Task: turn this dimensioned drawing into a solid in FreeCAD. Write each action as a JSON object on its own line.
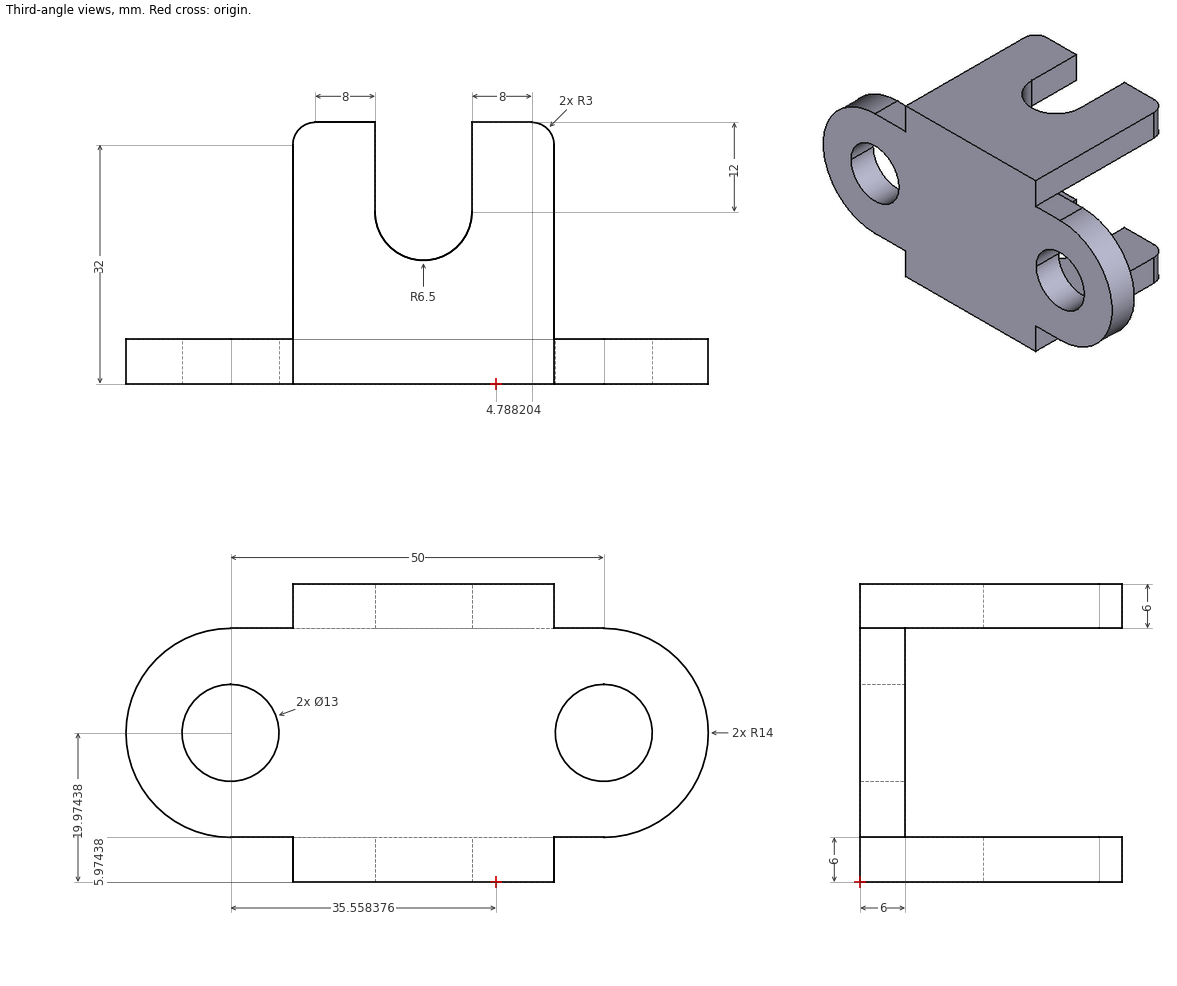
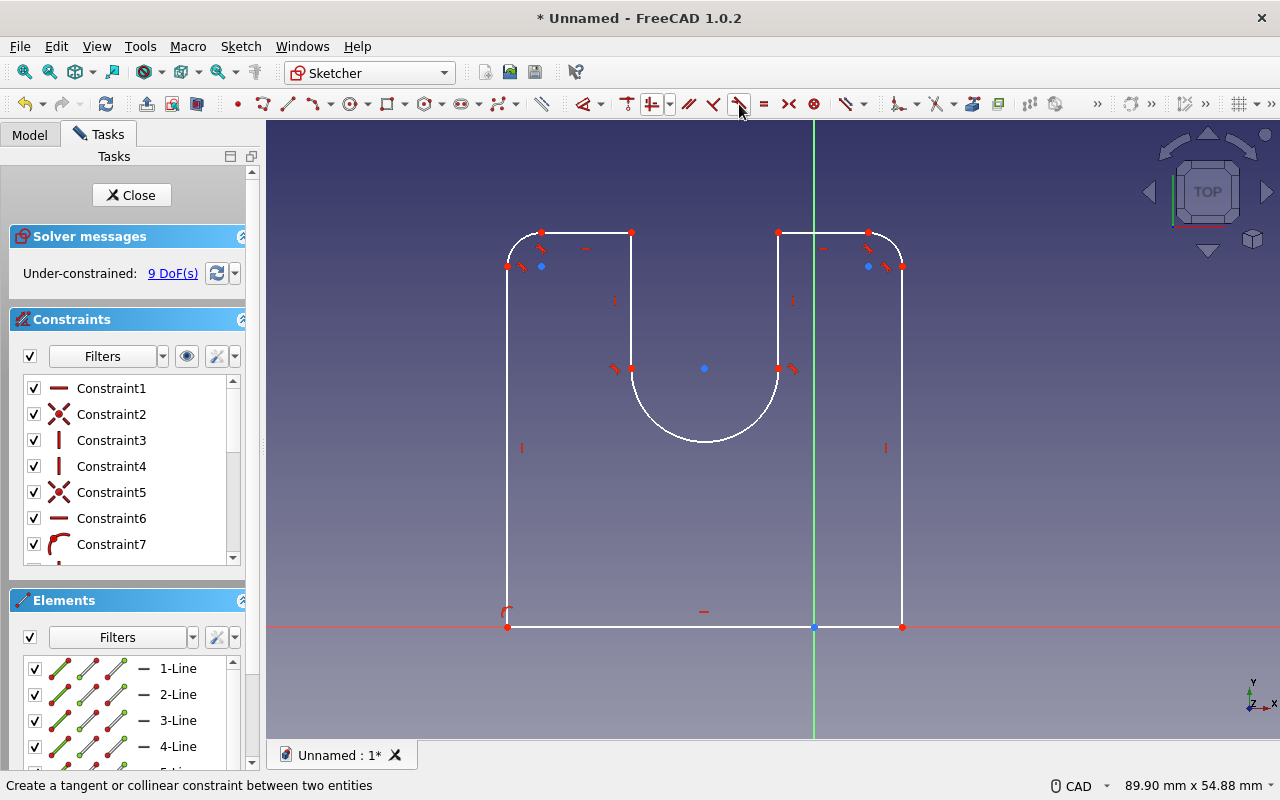
{"action": "left_click", "coordinate": [526, 237]}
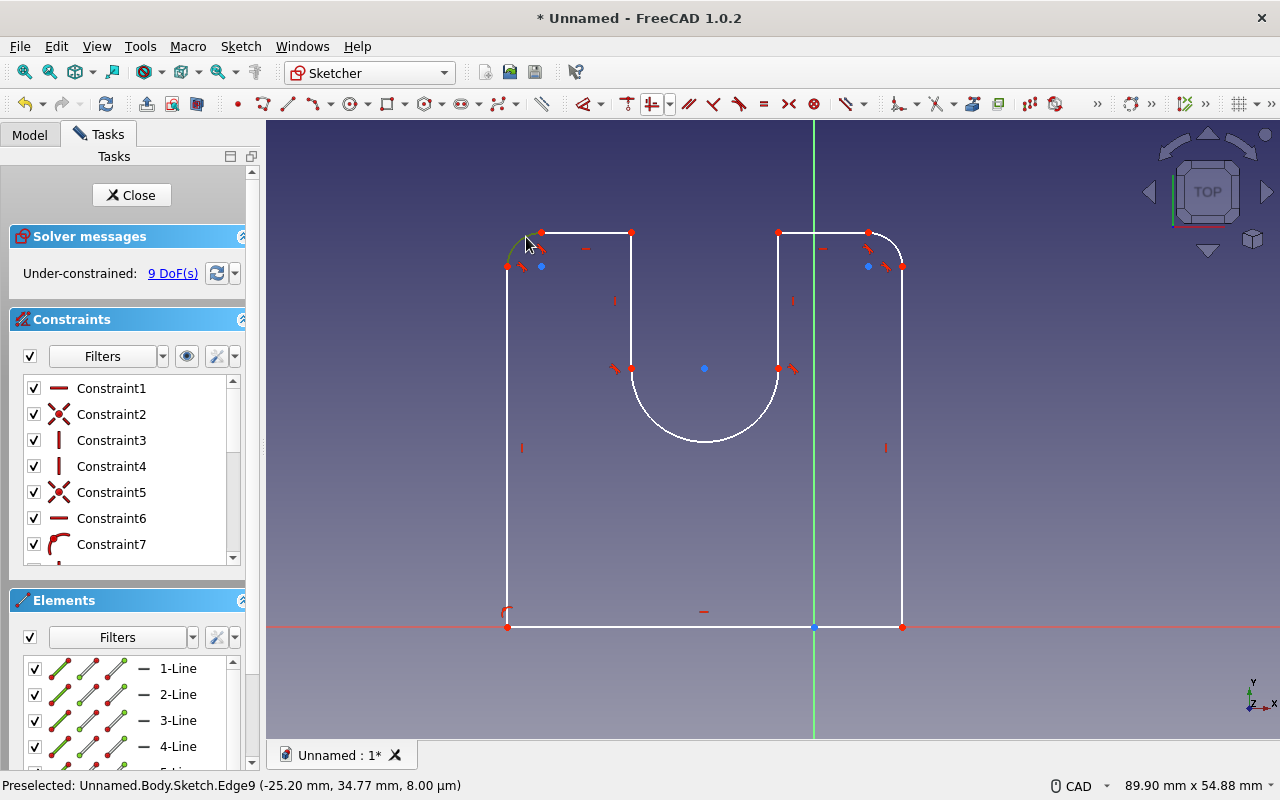
{"action": "left_click", "coordinate": [899, 252]}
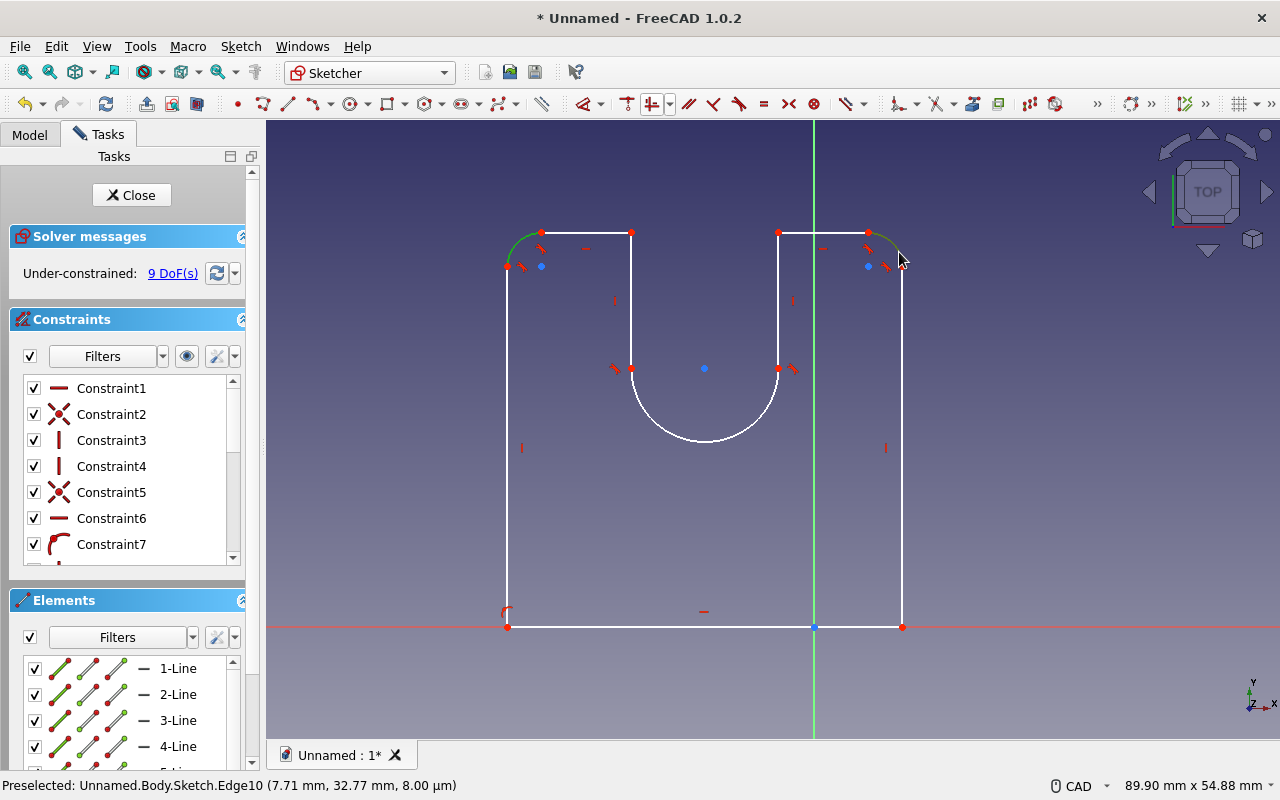
{"action": "left_click", "coordinate": [764, 104]}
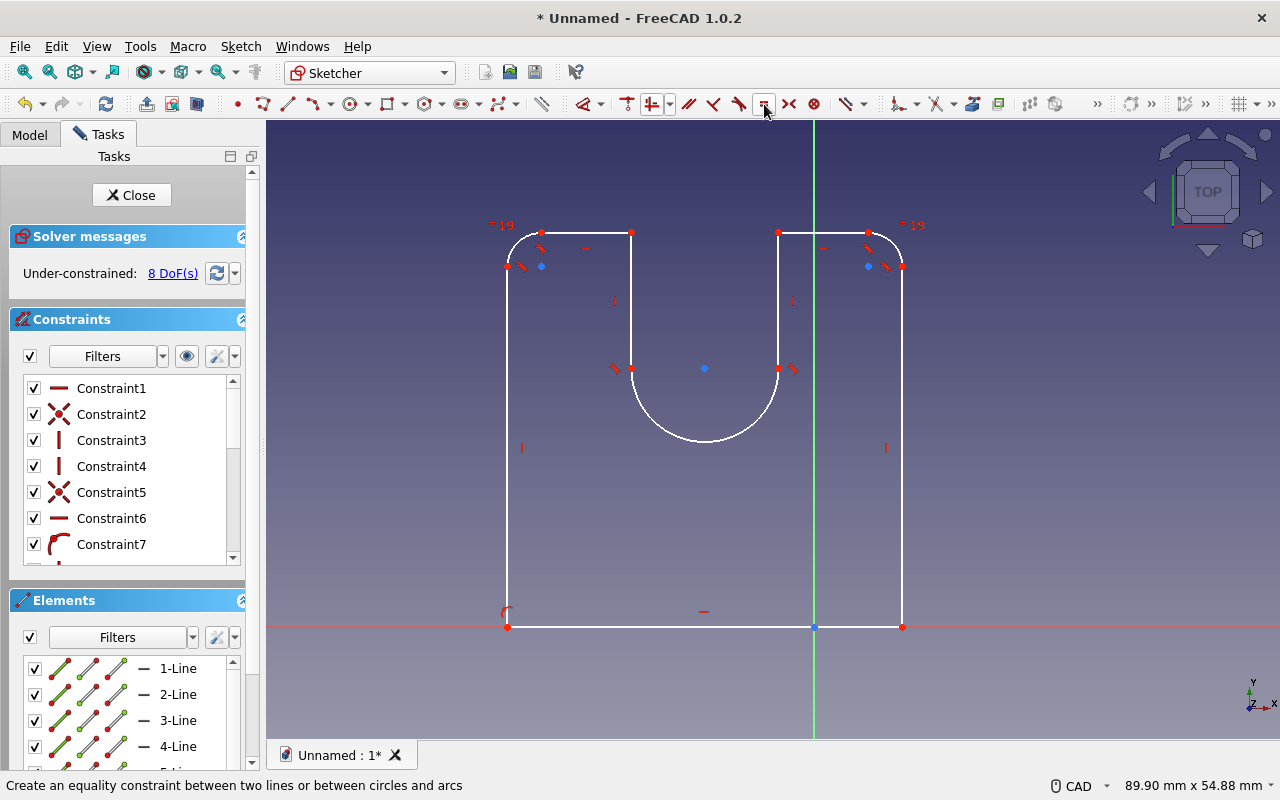
{"action": "left_click", "coordinate": [582, 104]}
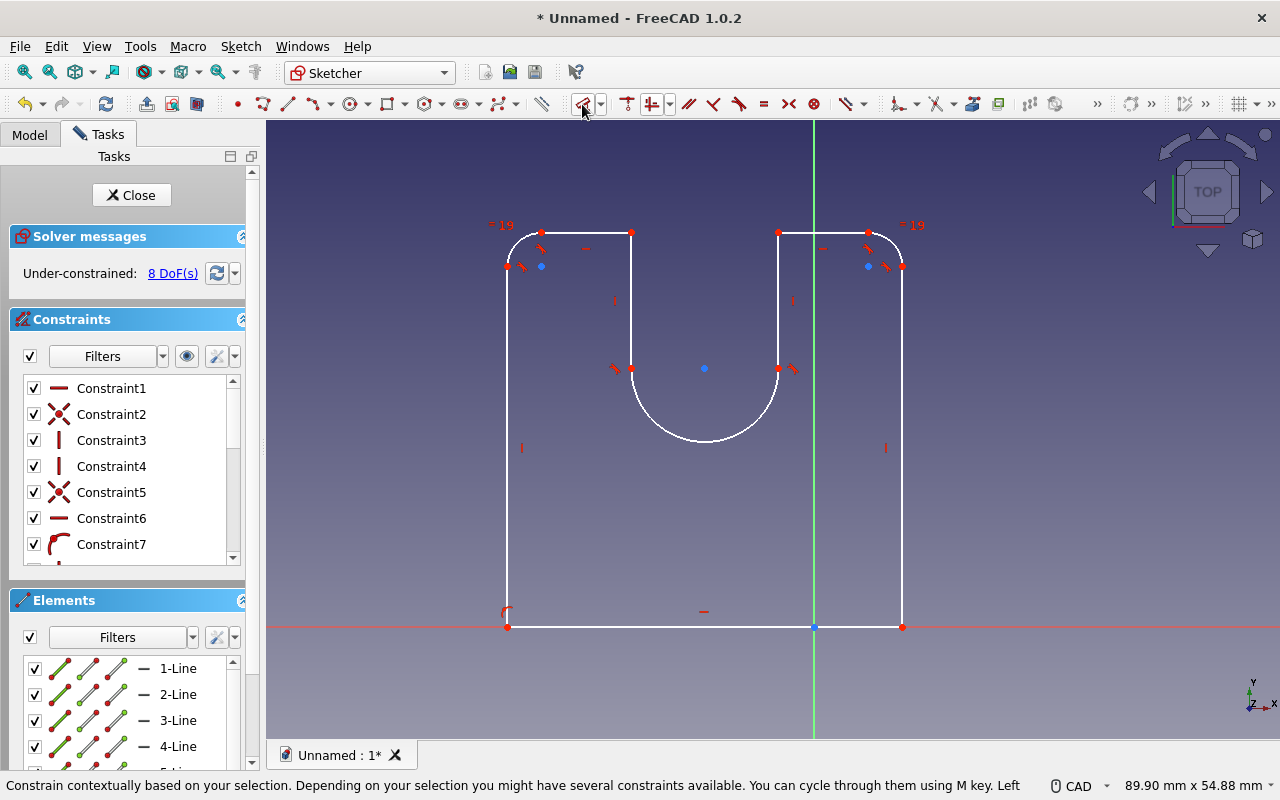
{"action": "left_click", "coordinate": [662, 428]}
{"action": "left_click", "coordinate": [643, 454]}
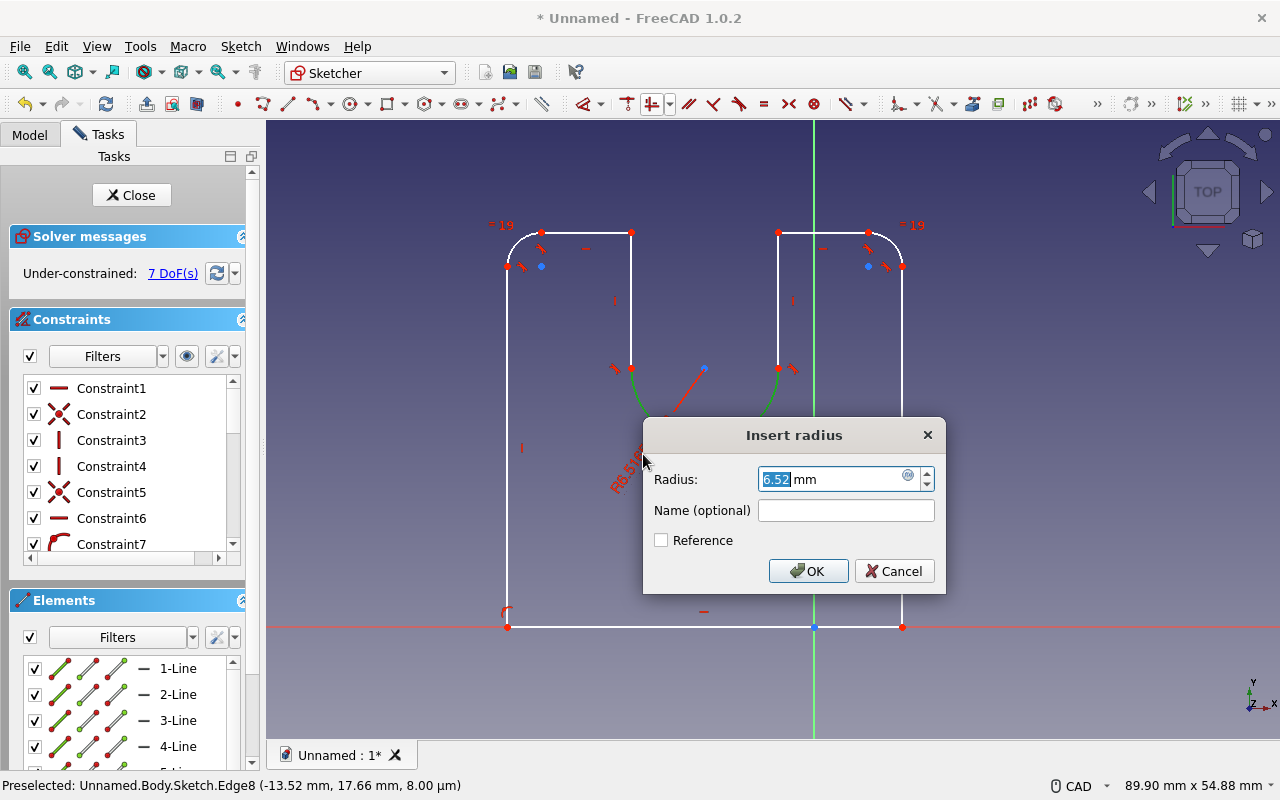
{"action": "type", "text": "6.5"}
{"action": "key", "text": "Return"}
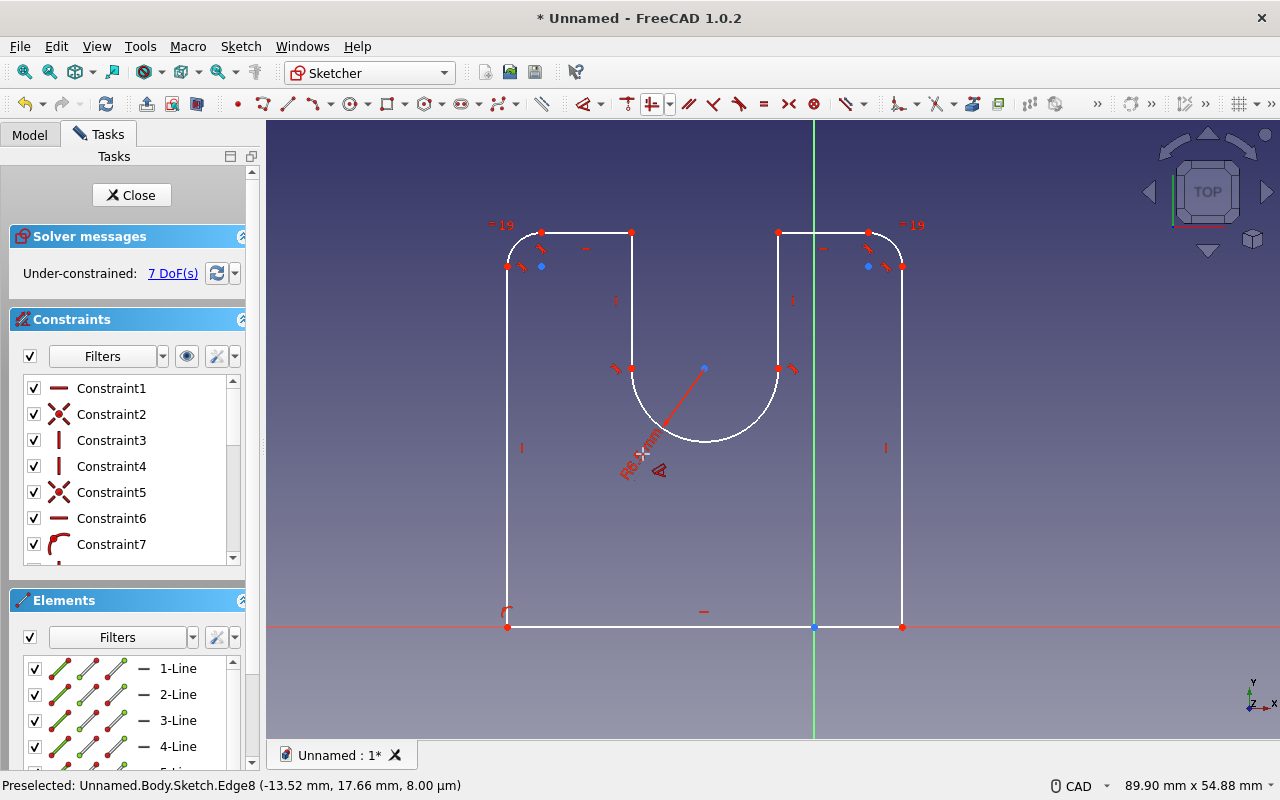
{"action": "left_click", "coordinate": [526, 237]}
{"action": "left_click", "coordinate": [511, 209]}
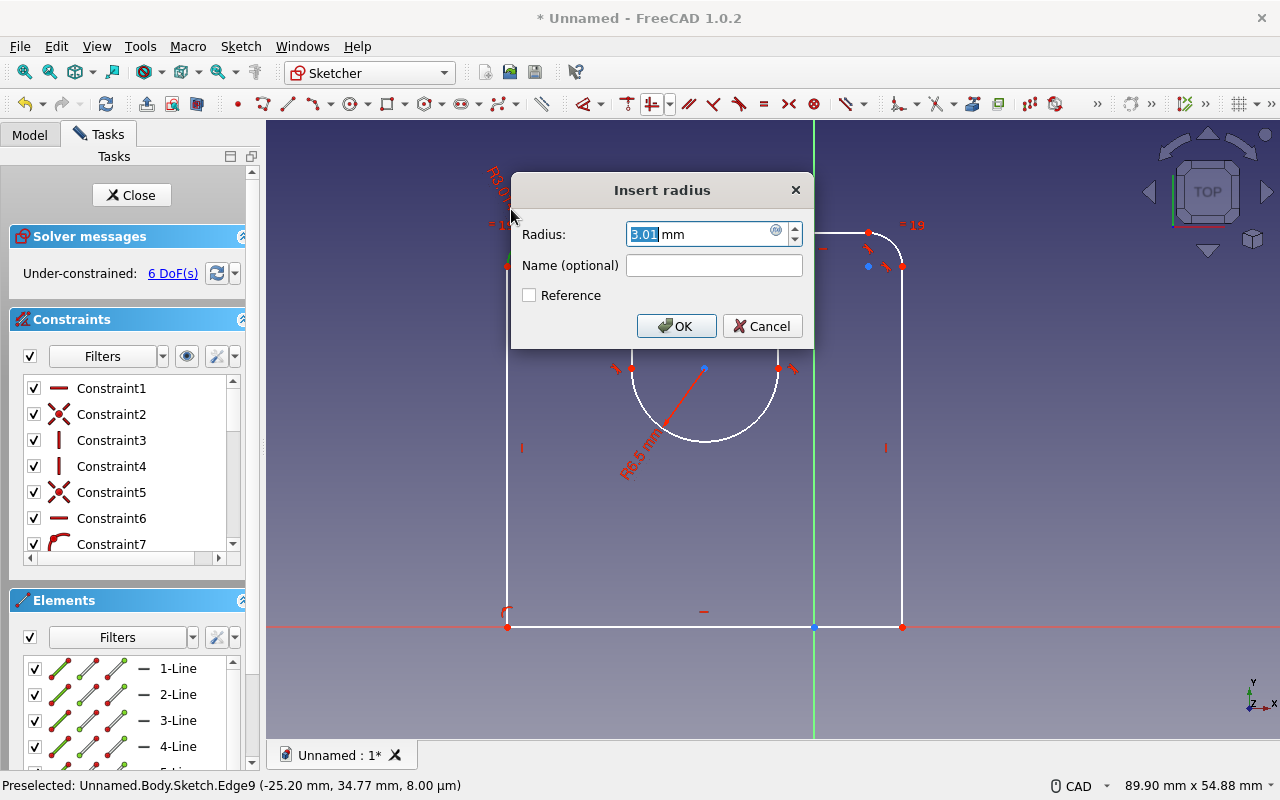
{"action": "type", "text": "3"}
{"action": "key", "text": "Return"}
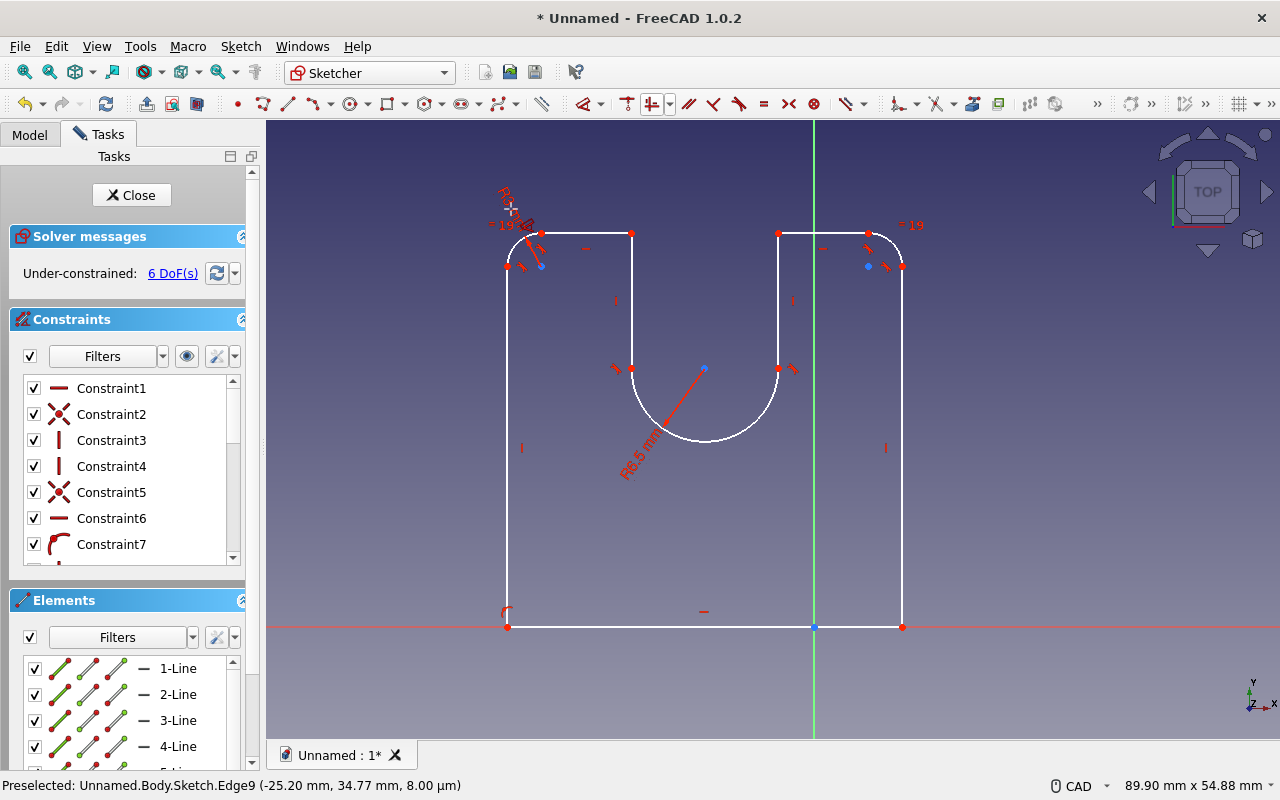
{"action": "left_click", "coordinate": [841, 233]}
{"action": "left_click", "coordinate": [844, 199]}